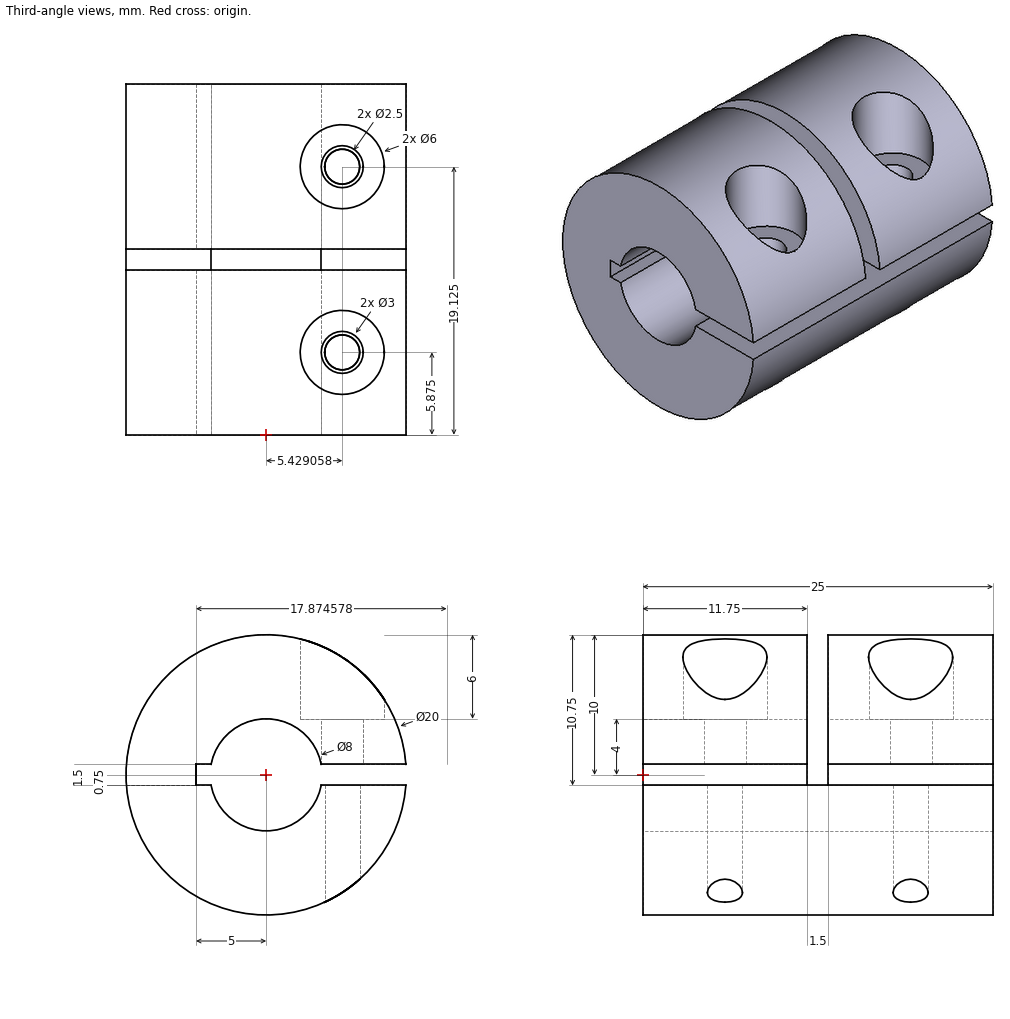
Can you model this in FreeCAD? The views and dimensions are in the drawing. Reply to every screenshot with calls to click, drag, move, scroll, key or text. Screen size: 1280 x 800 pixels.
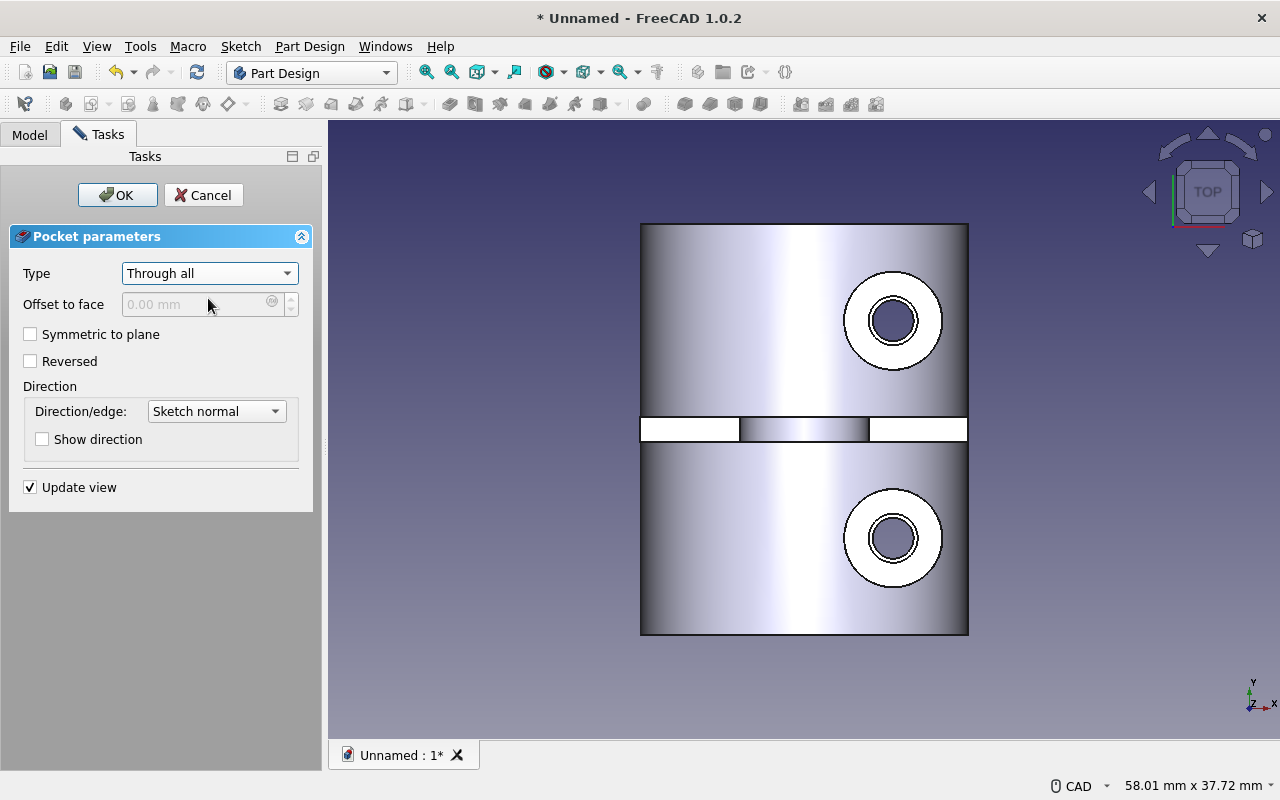
click(118, 195)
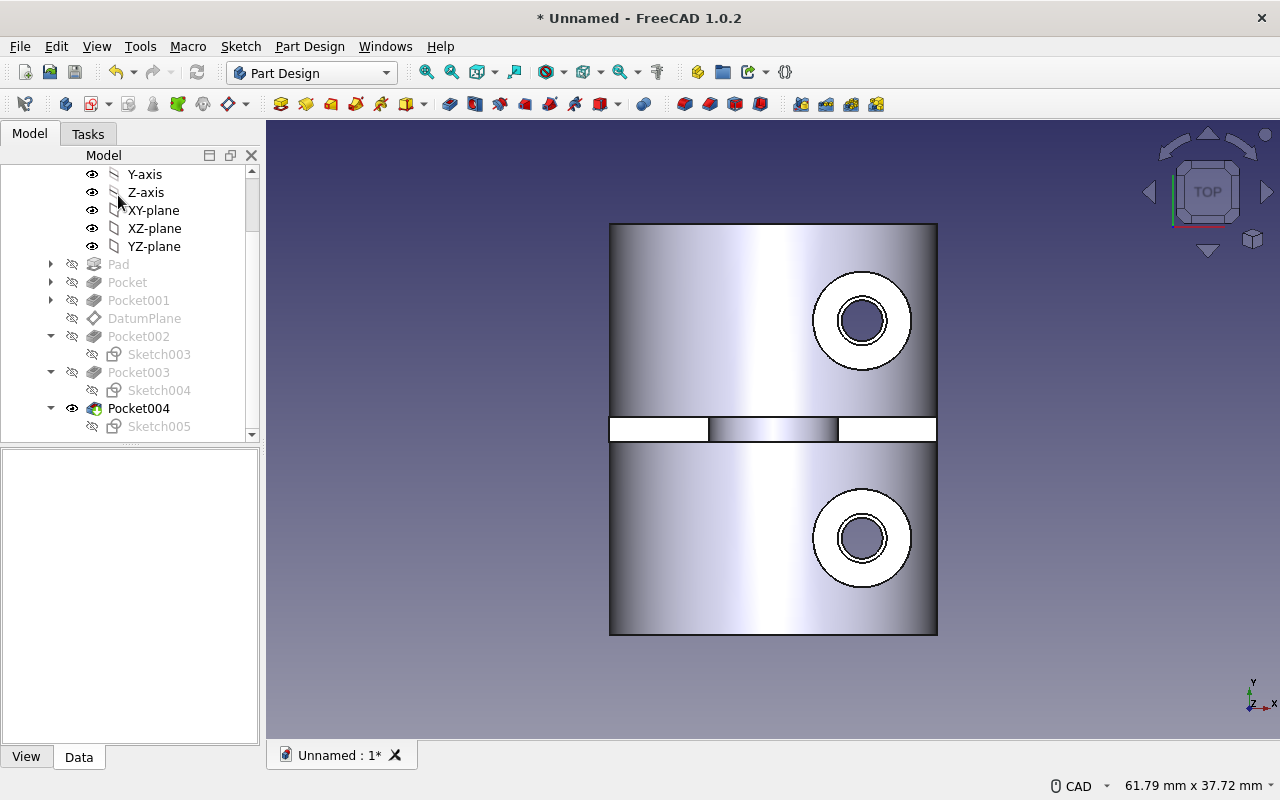
key(0)